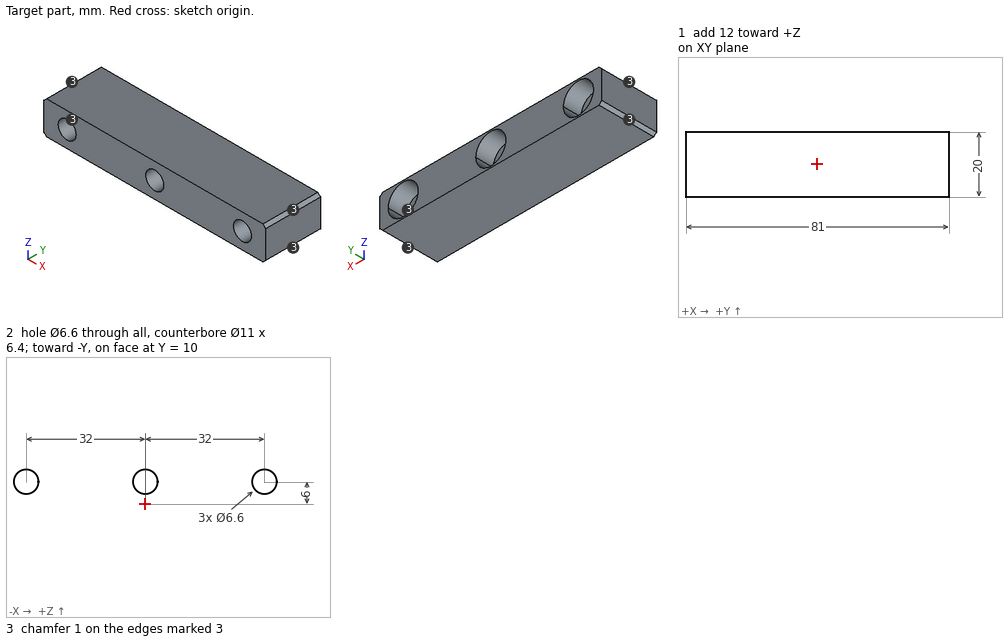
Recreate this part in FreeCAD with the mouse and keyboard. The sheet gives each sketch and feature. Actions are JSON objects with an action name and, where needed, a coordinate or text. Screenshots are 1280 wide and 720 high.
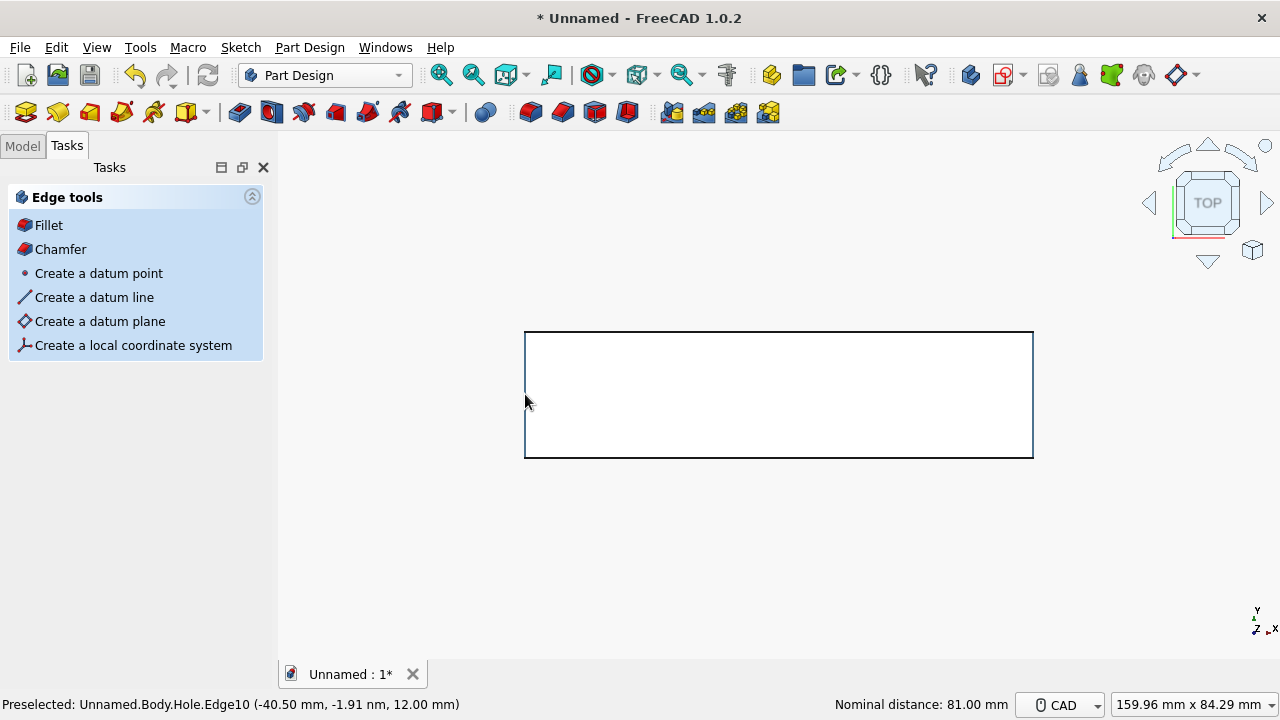
{"action": "key", "text": "1"}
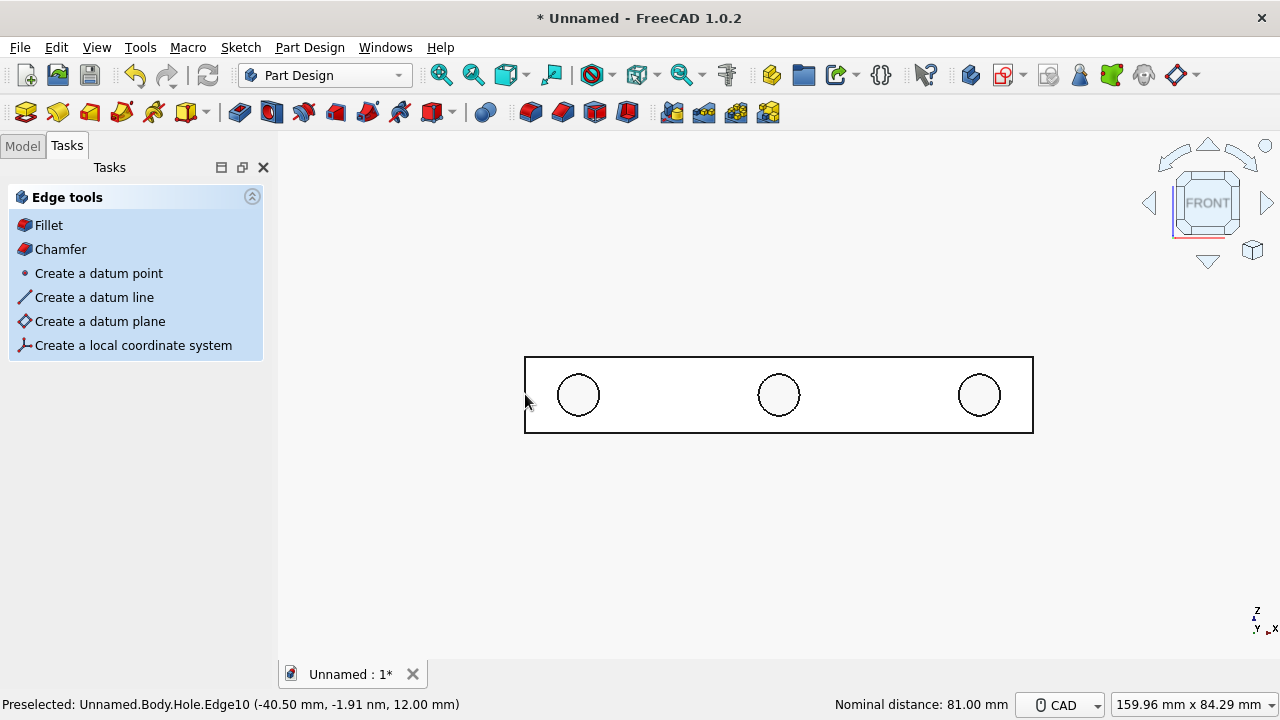
{"action": "key", "text": "3"}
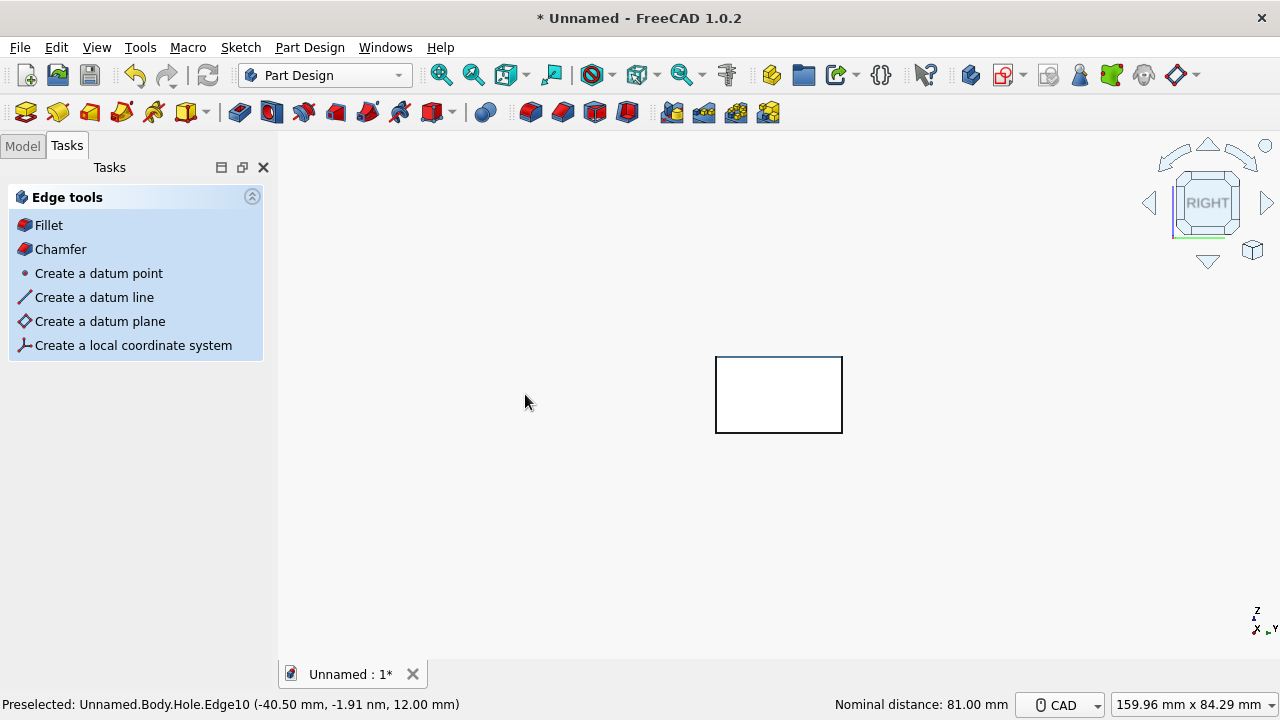
{"action": "left_click", "coordinate": [442, 76]}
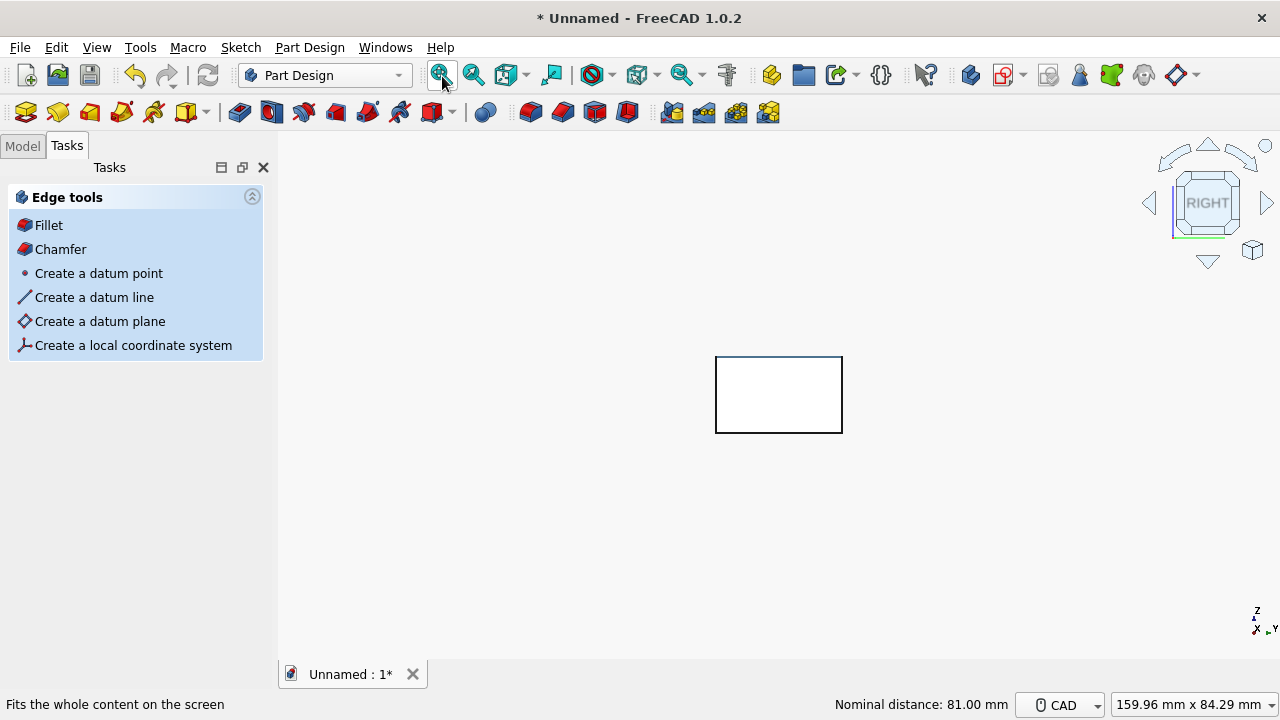
{"action": "left_click", "coordinate": [779, 432], "text": "ctrl"}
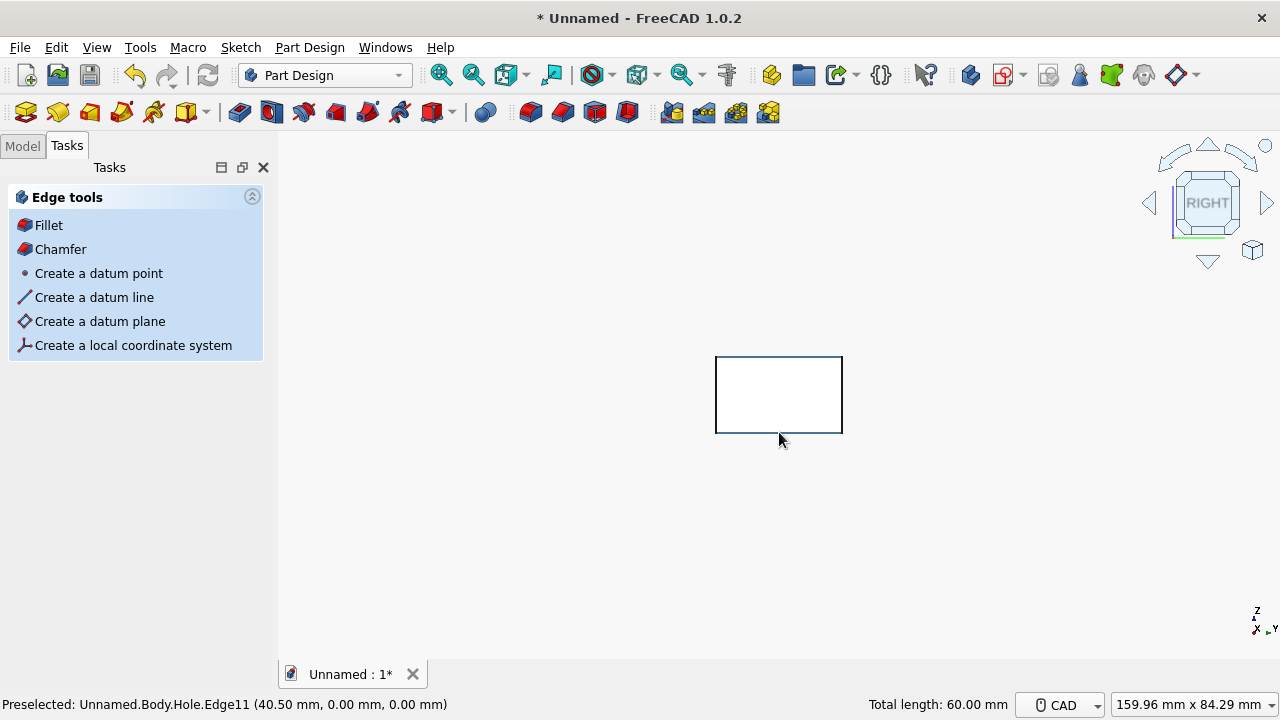
{"action": "key", "text": "5"}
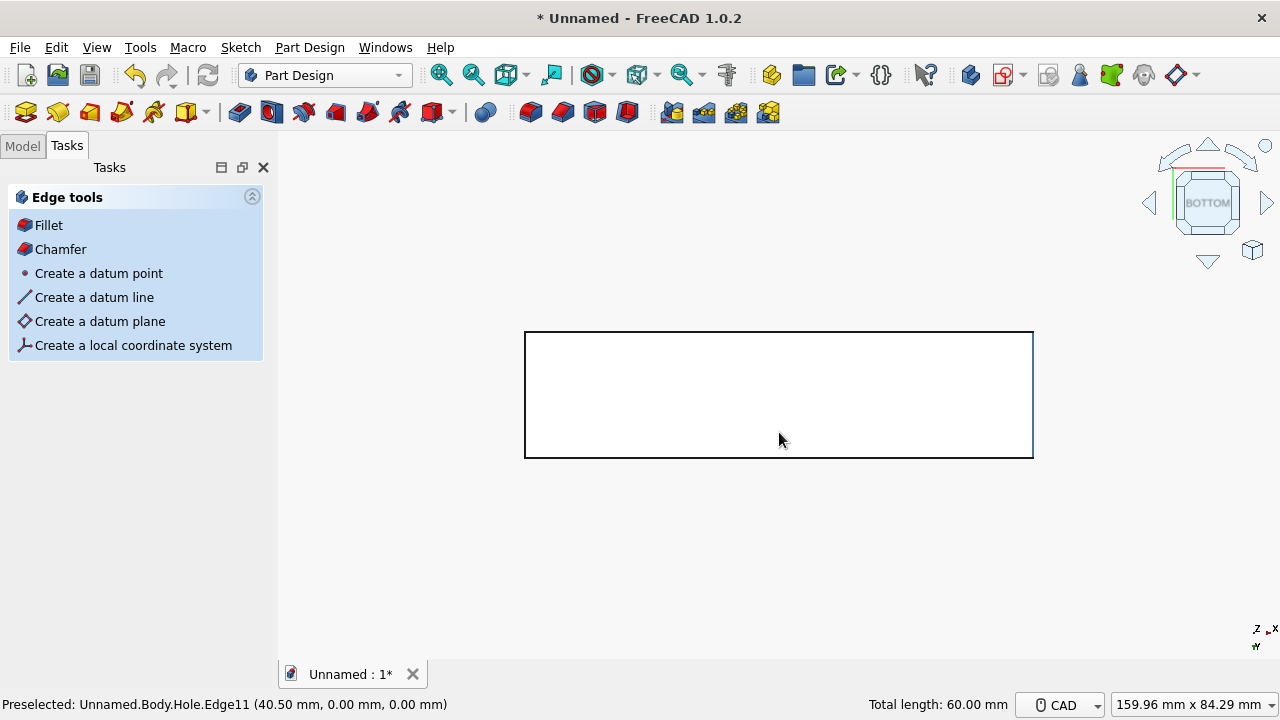
{"action": "left_click", "coordinate": [525, 394], "text": "ctrl"}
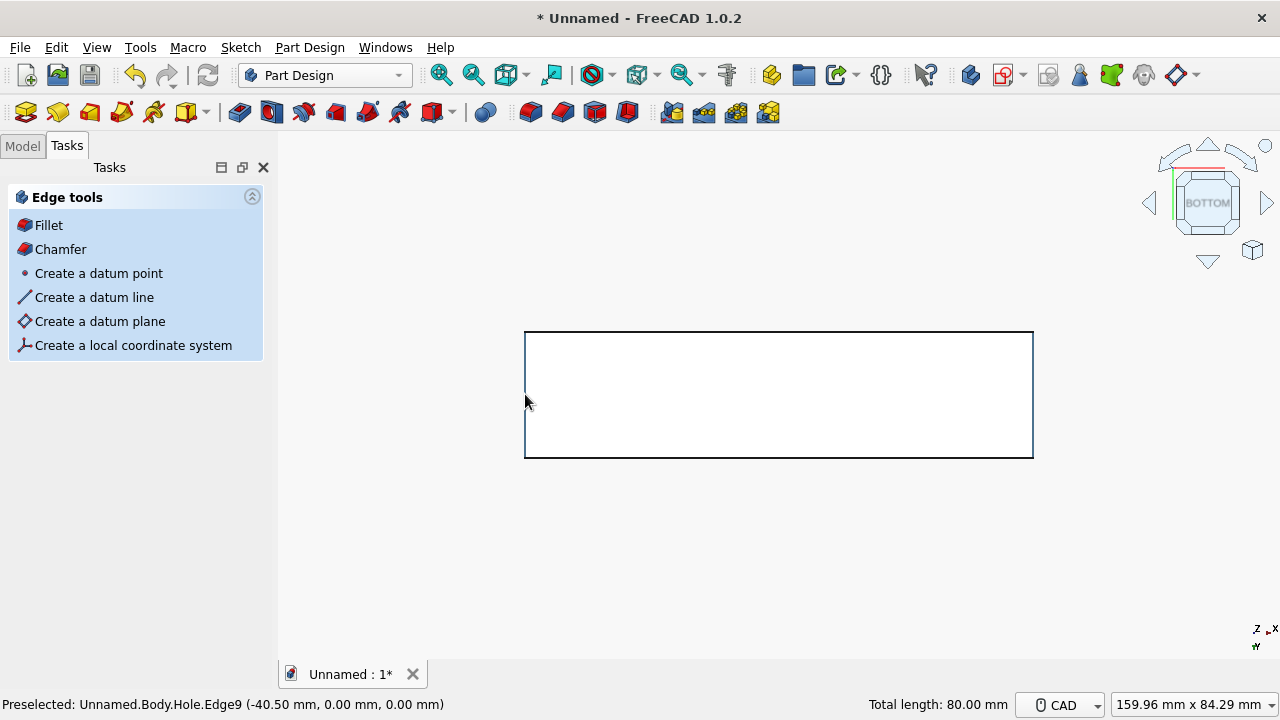
{"action": "left_click", "coordinate": [564, 112]}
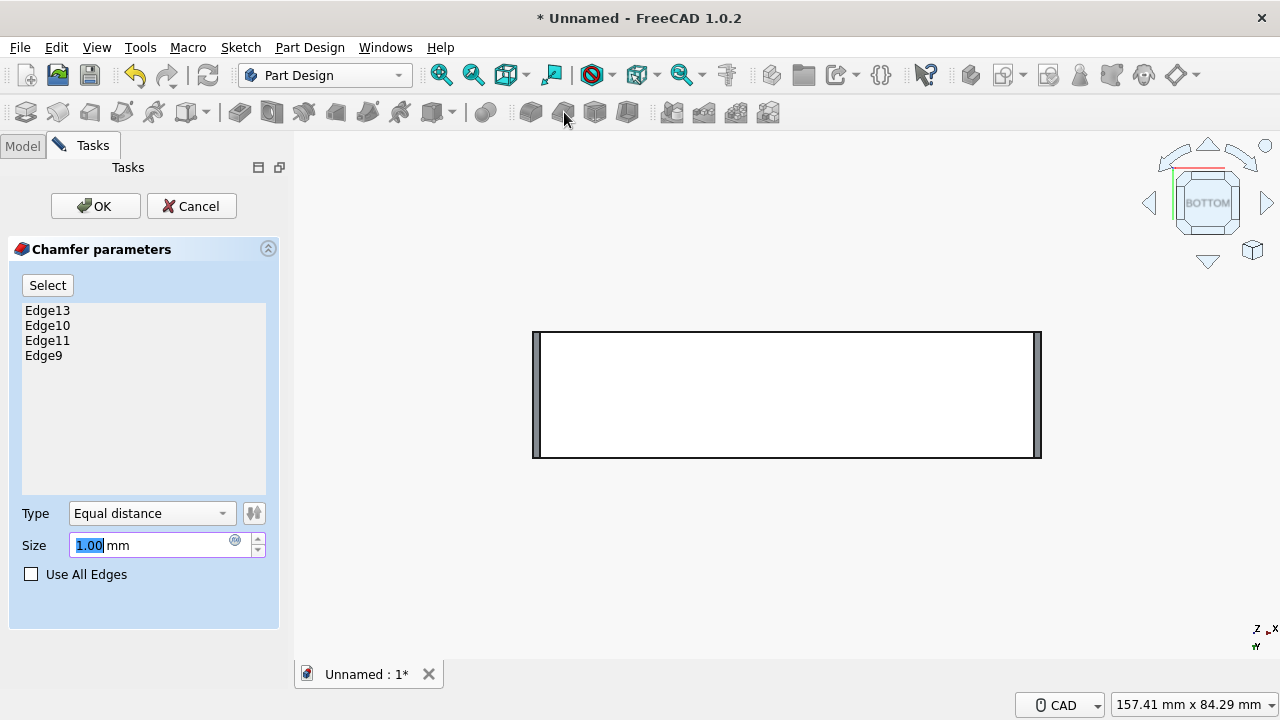
{"action": "type", "text": "1"}
{"action": "key", "text": "Tab"}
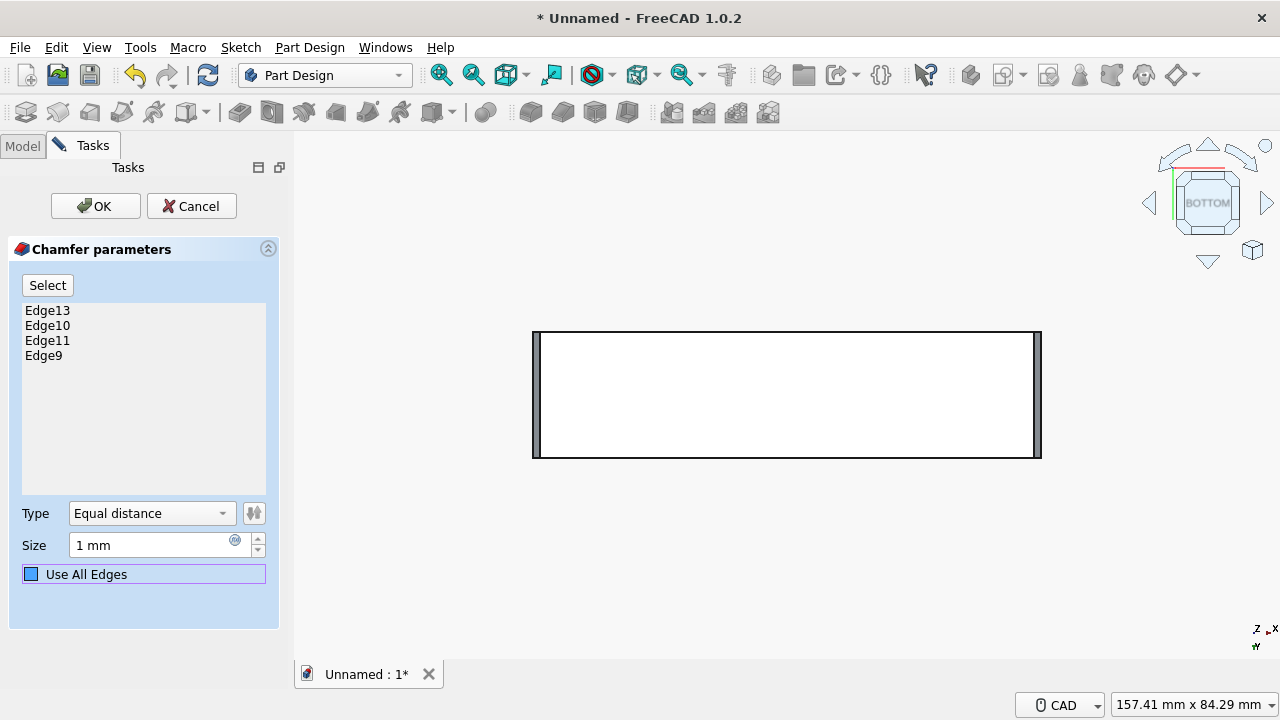
{"action": "left_click", "coordinate": [96, 206]}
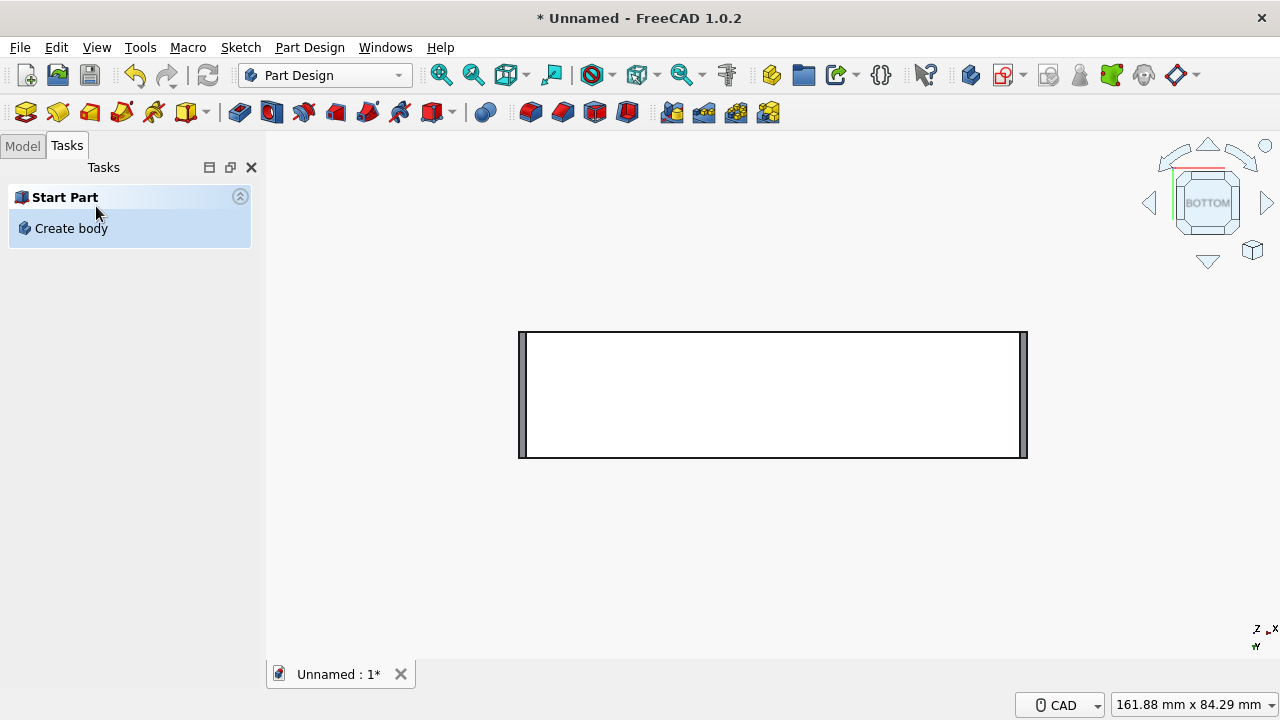
{"action": "key", "text": "0"}